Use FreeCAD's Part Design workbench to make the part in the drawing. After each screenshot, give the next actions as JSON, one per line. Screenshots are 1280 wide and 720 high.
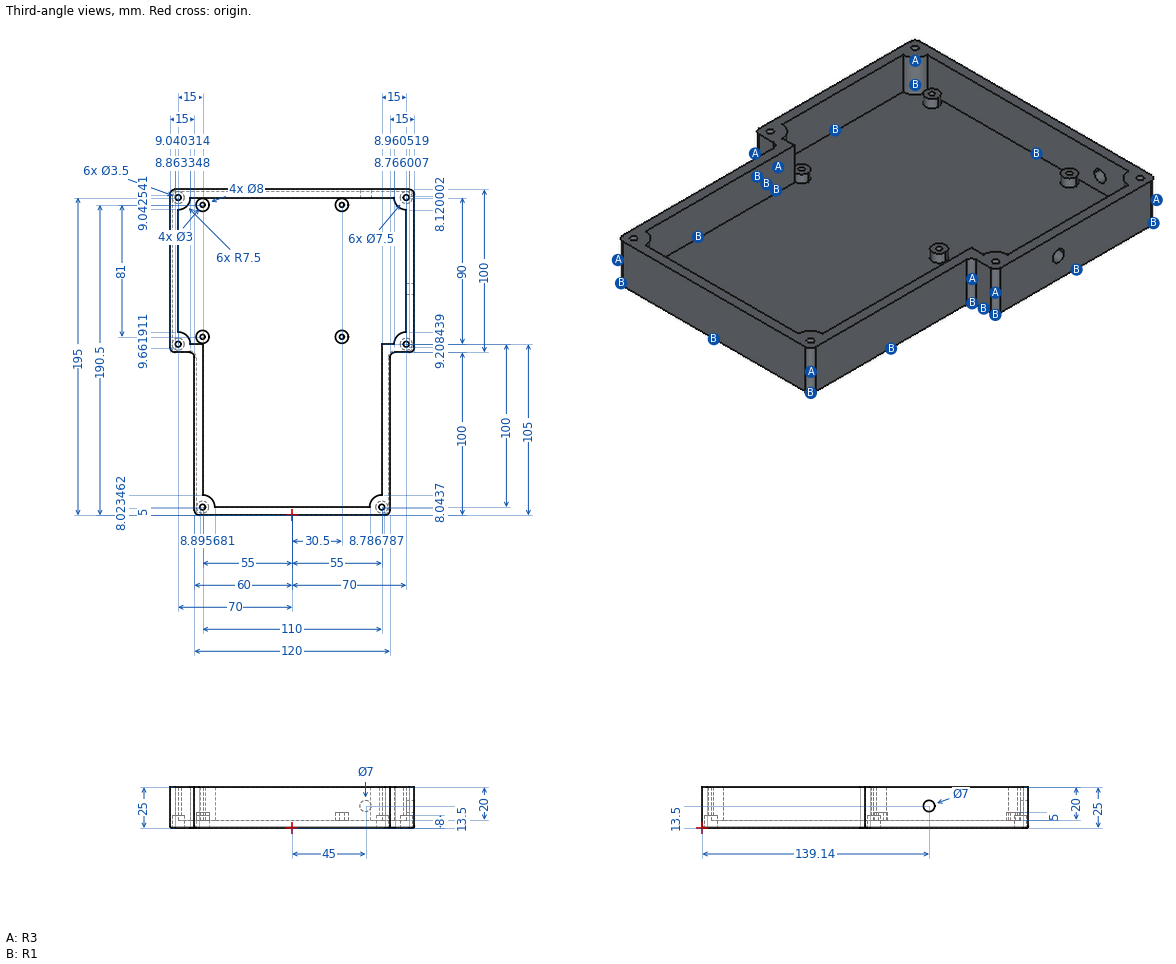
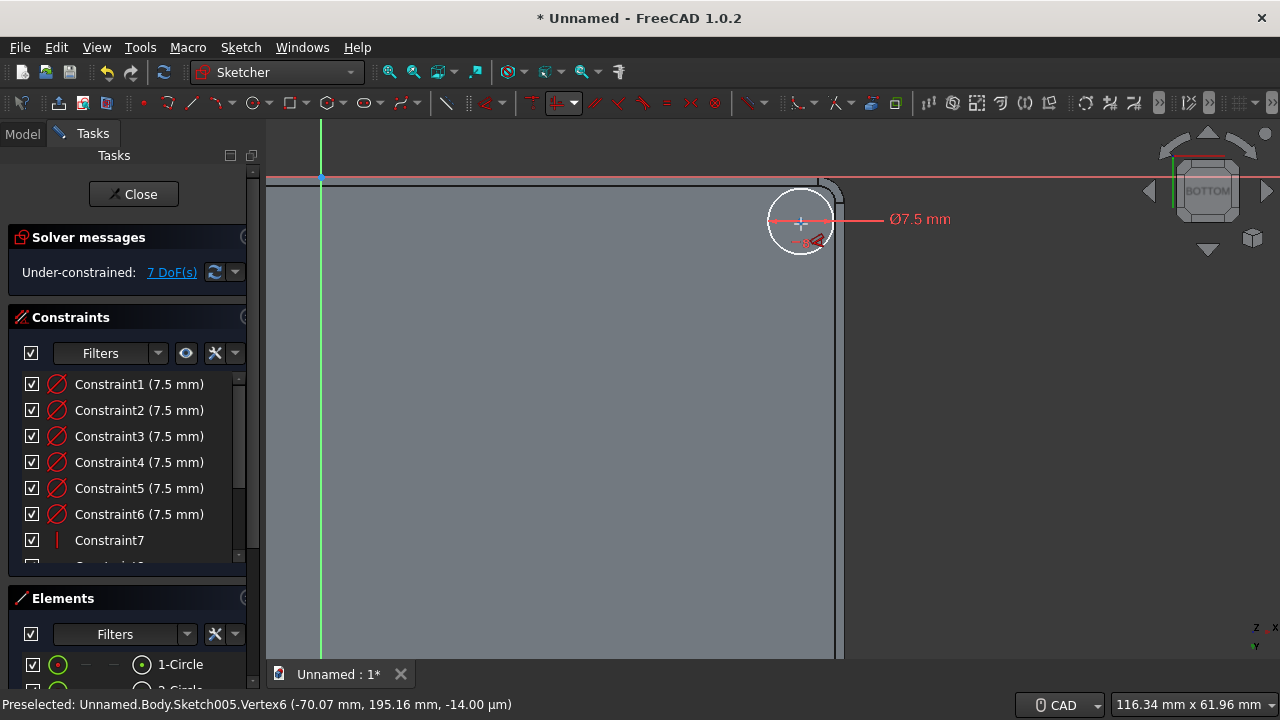
{"action": "left_click", "coordinate": [801, 221]}
{"action": "left_click", "coordinate": [859, 199]}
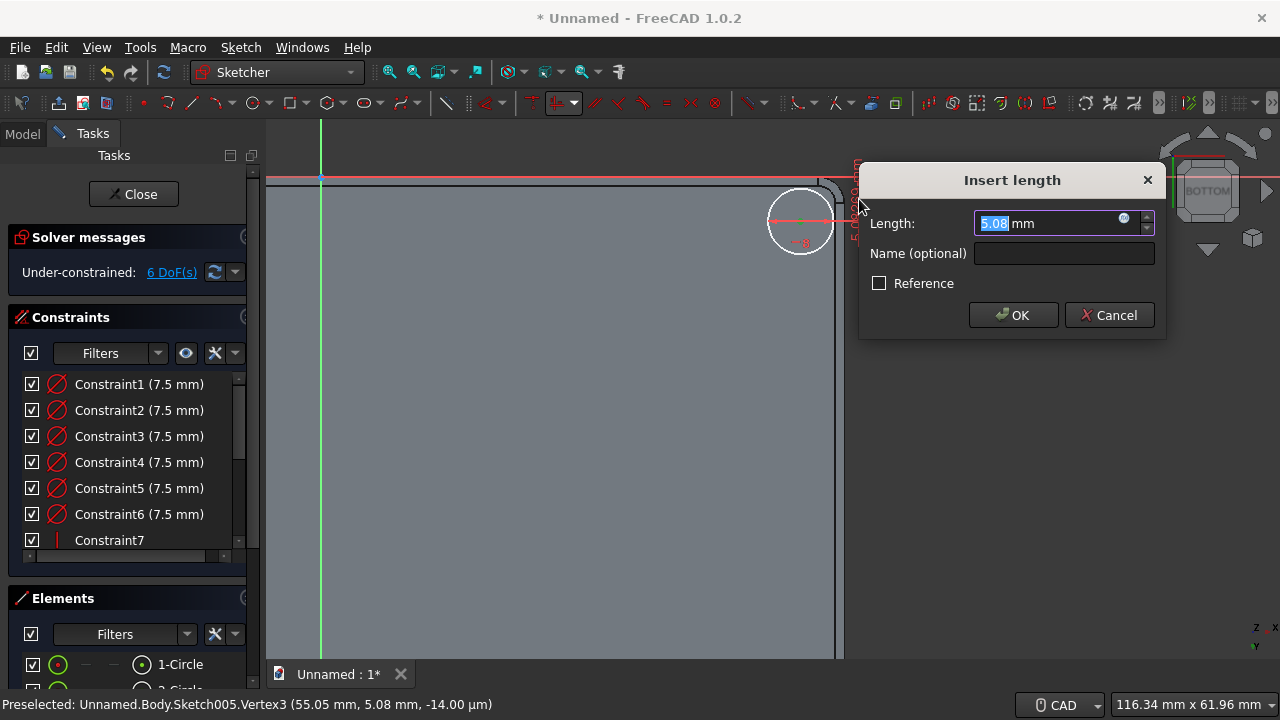
{"action": "type", "text": "5"}
{"action": "key", "text": "Return"}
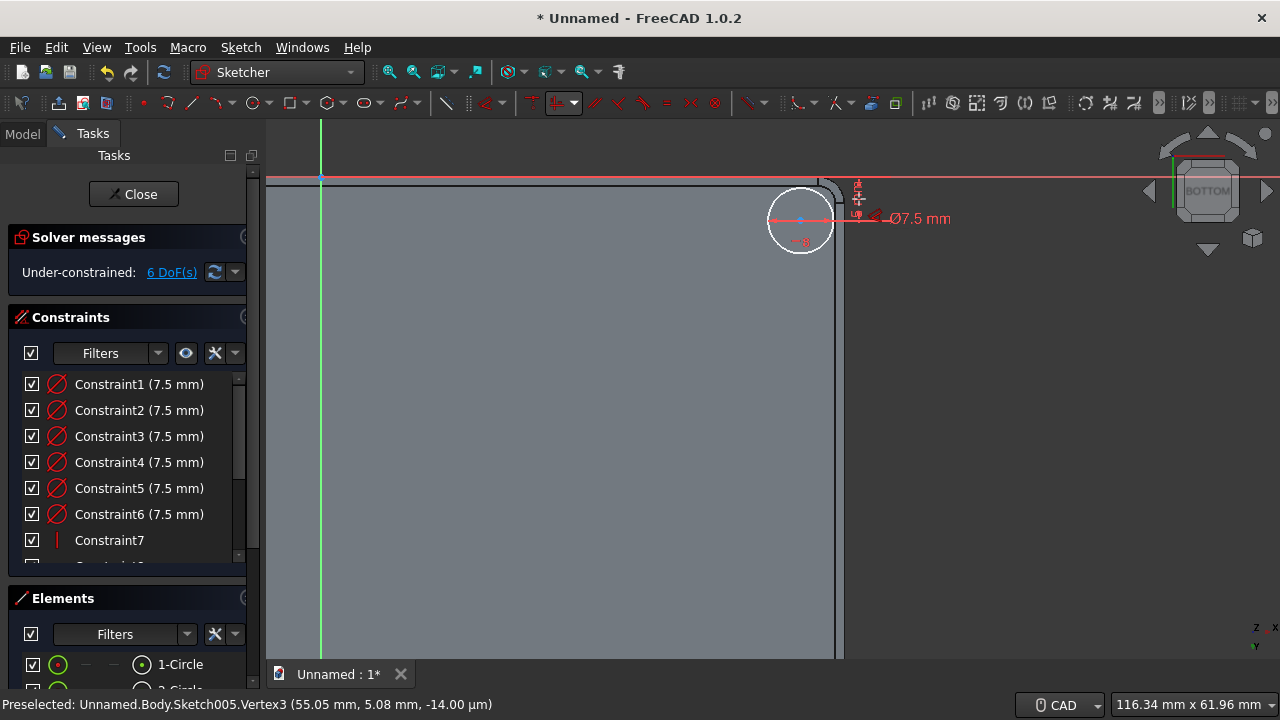
{"action": "scroll", "coordinate": [801, 223], "scroll_direction": "down", "scroll_amount": 8}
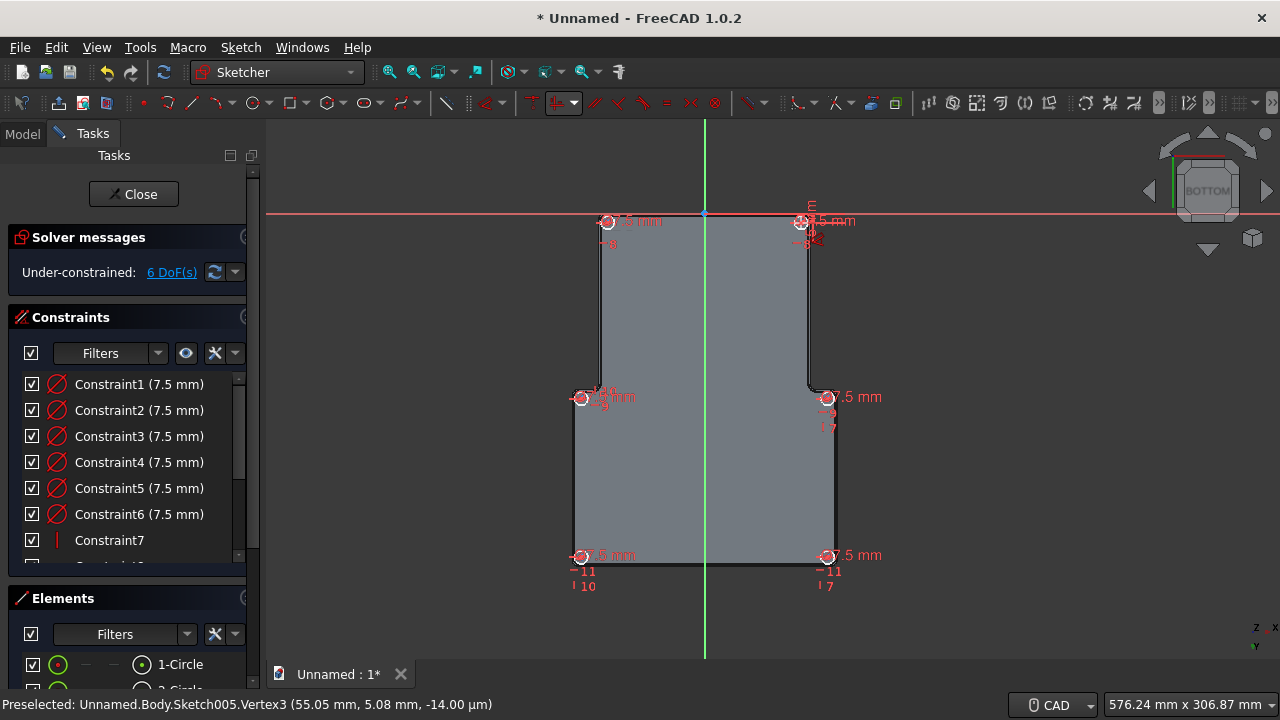
{"action": "left_click", "coordinate": [828, 557]}
{"action": "left_click", "coordinate": [766, 180]}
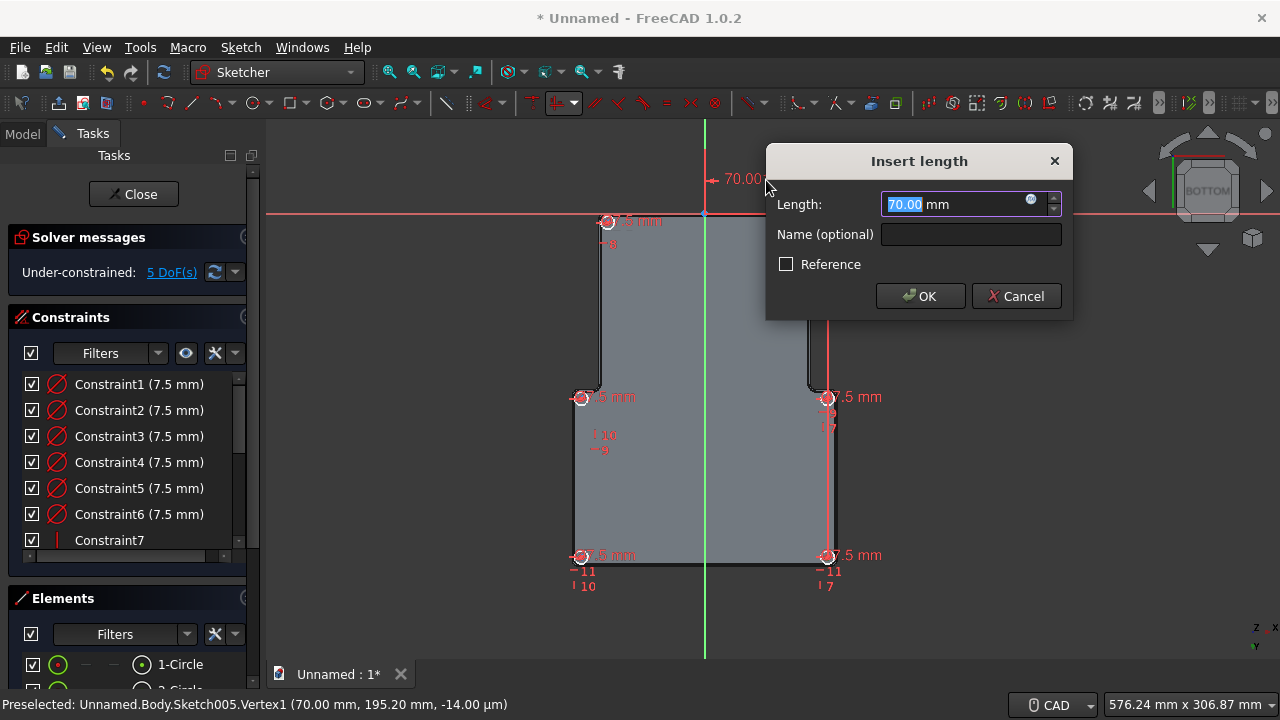
{"action": "type", "text": "70"}
{"action": "key", "text": "Return"}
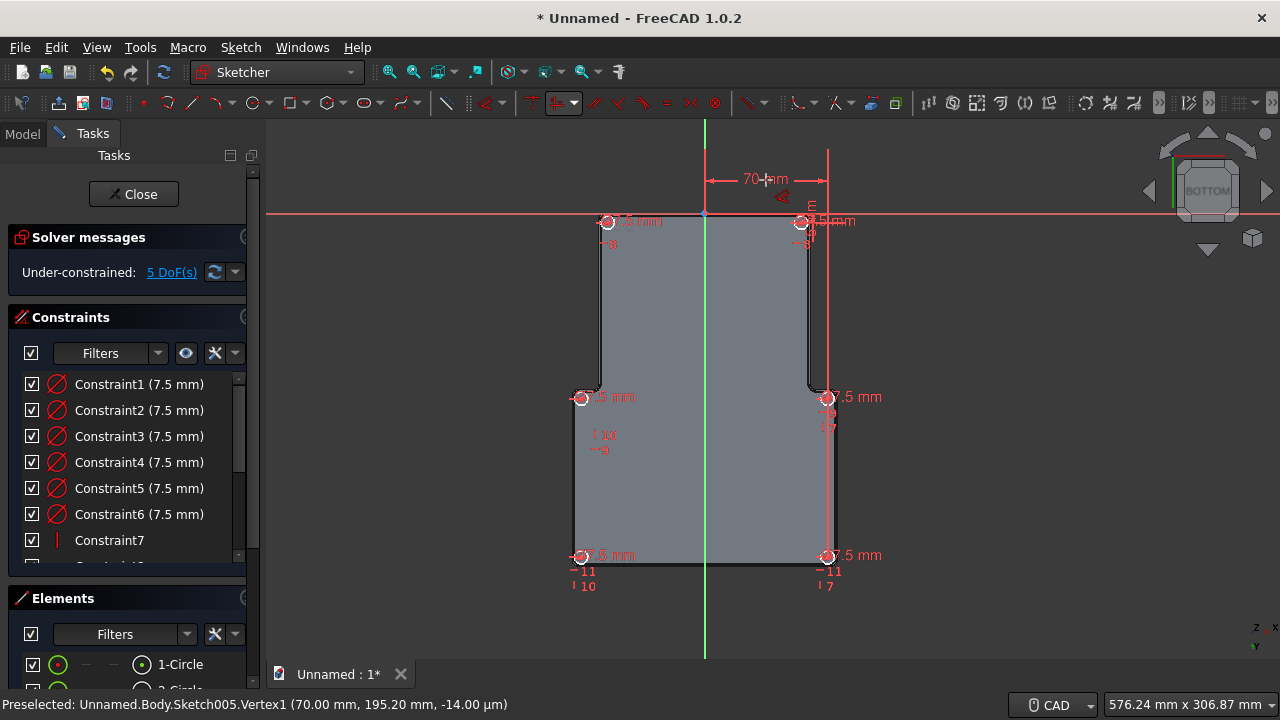
{"action": "left_click", "coordinate": [801, 223]}
{"action": "left_click", "coordinate": [753, 257]}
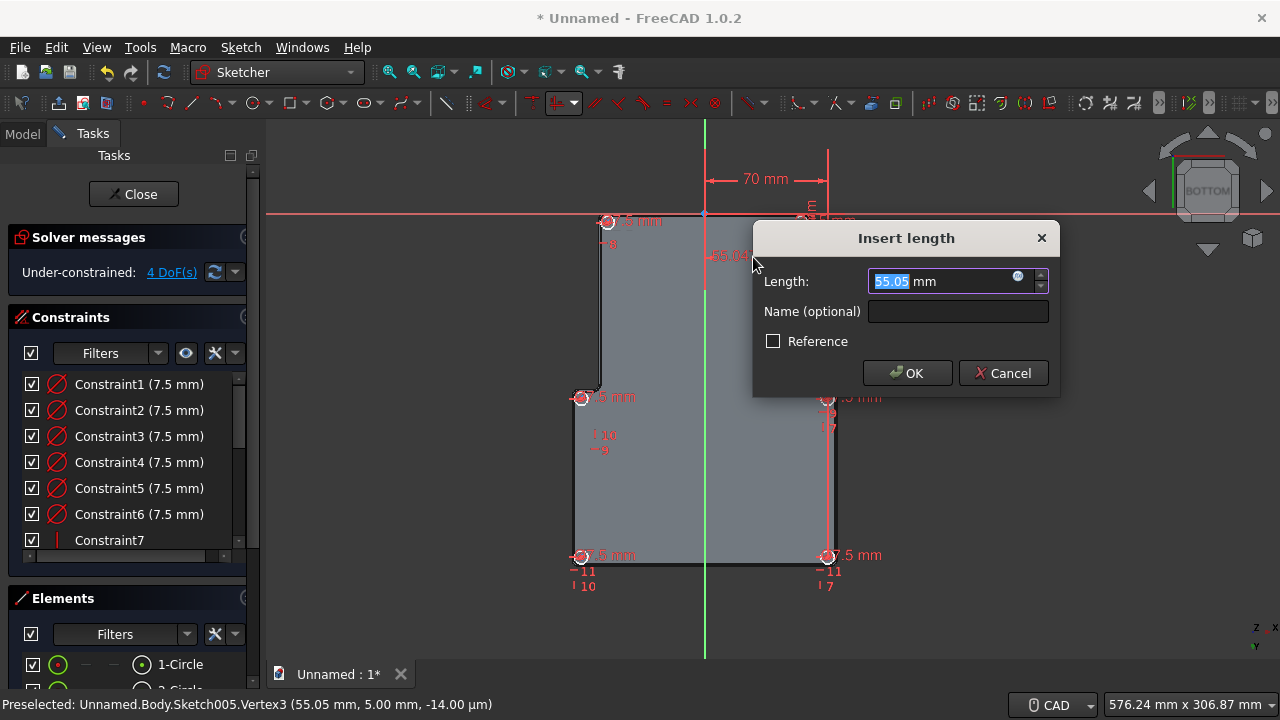
{"action": "type", "text": "55"}
{"action": "key", "text": "Return"}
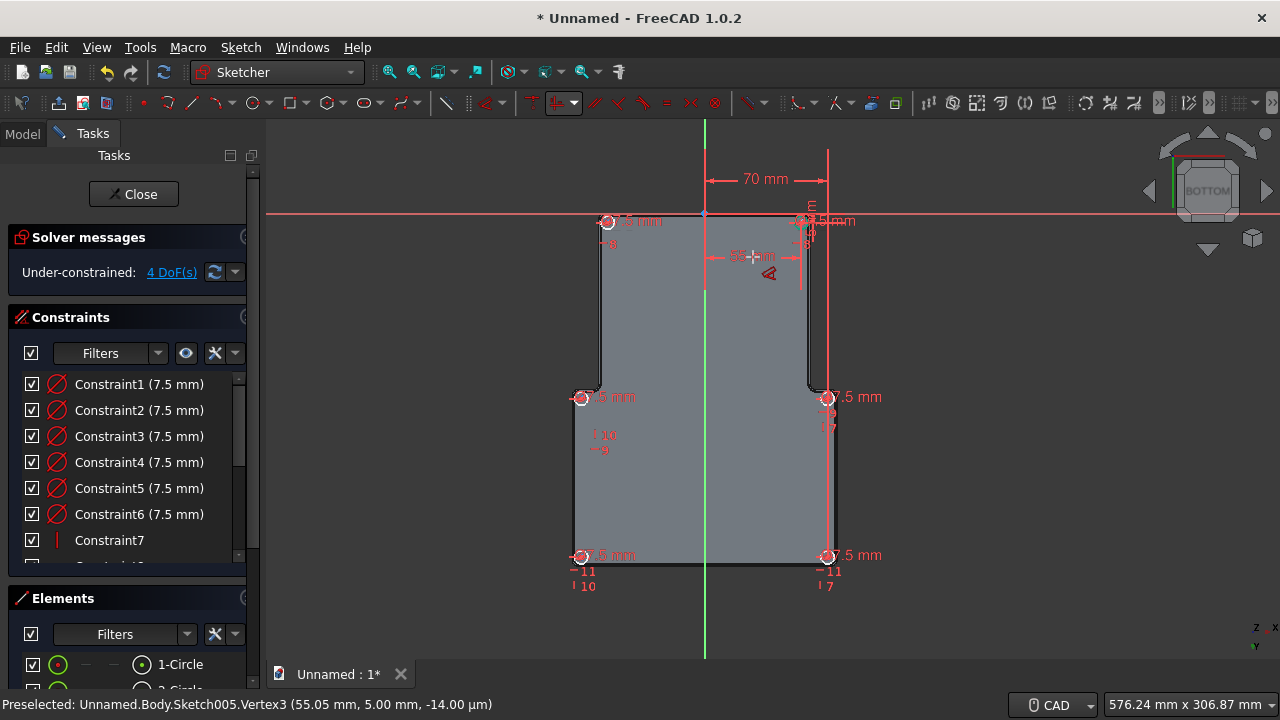
{"action": "left_click", "coordinate": [608, 223]}
{"action": "left_click", "coordinate": [656, 180]}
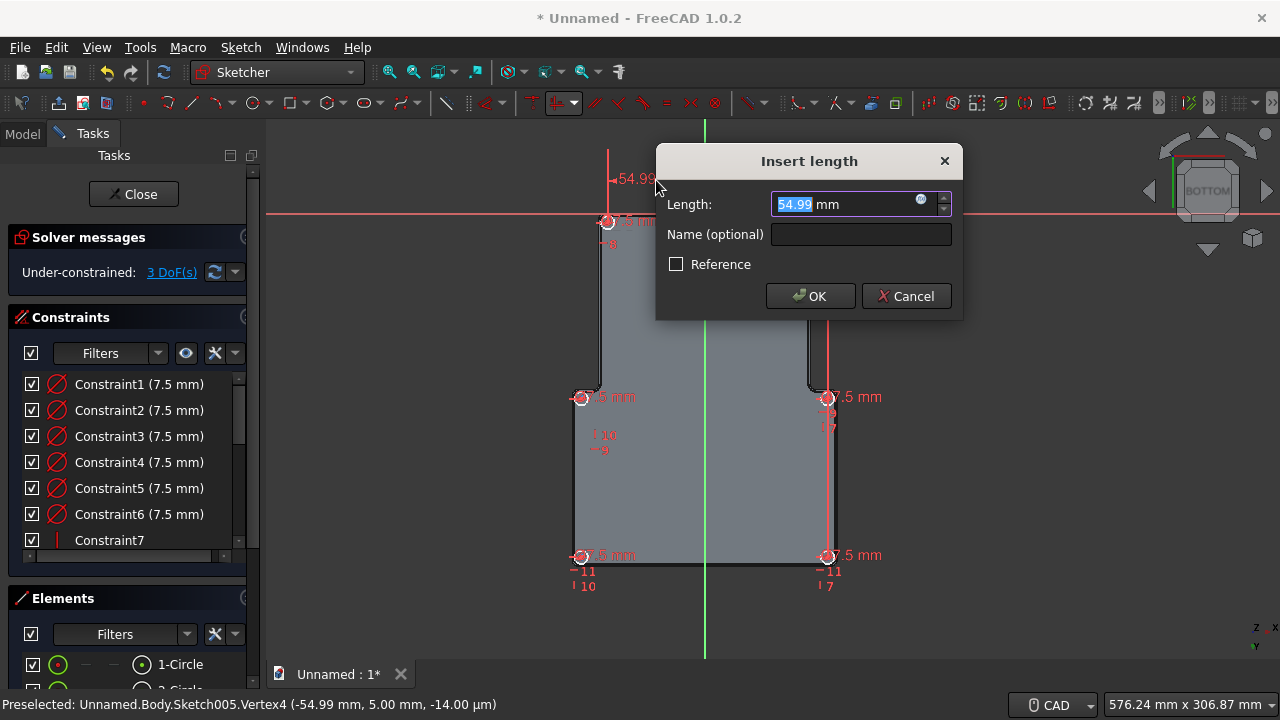
{"action": "type", "text": "55"}
{"action": "key", "text": "Return"}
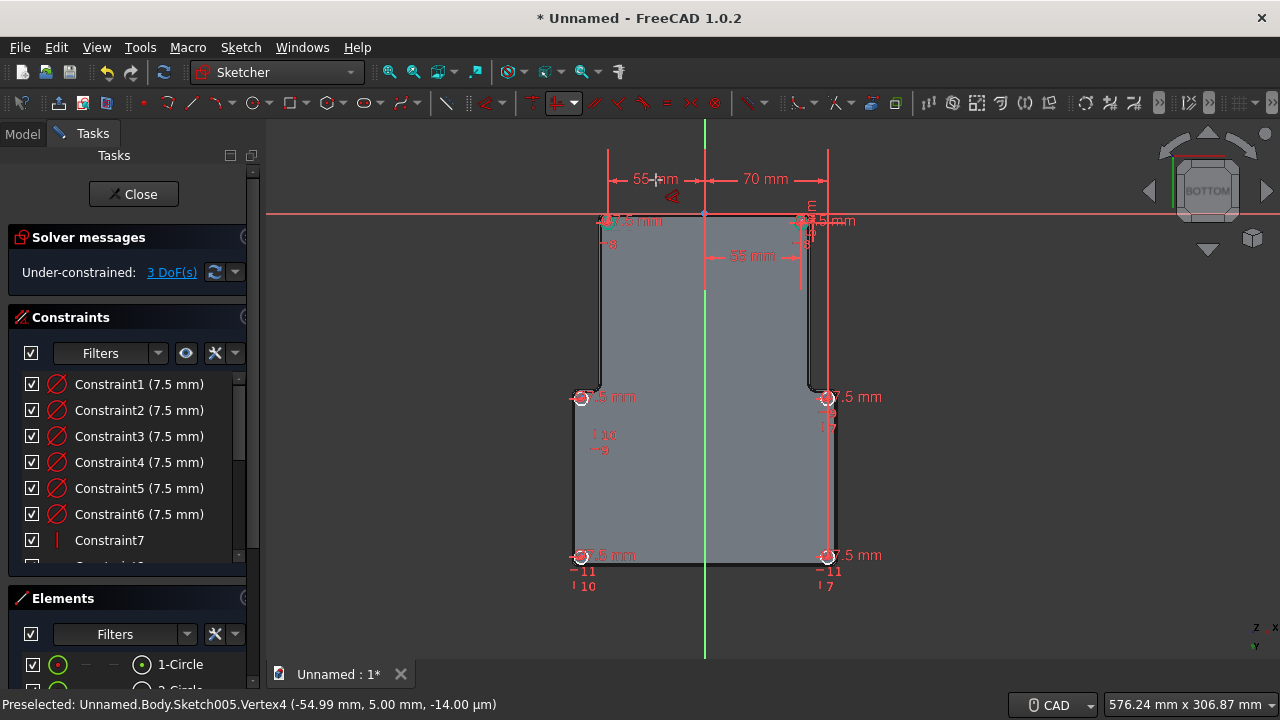
{"action": "left_click", "coordinate": [581, 399]}
{"action": "left_click", "coordinate": [643, 433]}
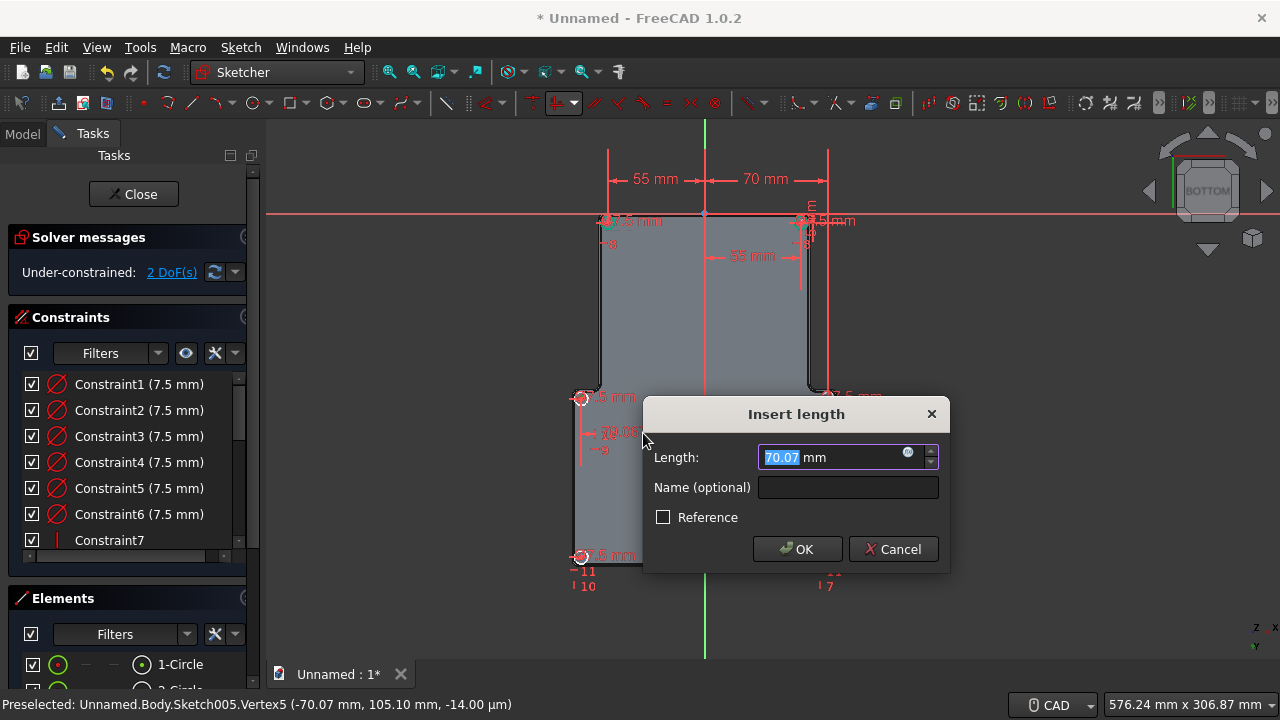
{"action": "type", "text": "70"}
{"action": "key", "text": "Return"}